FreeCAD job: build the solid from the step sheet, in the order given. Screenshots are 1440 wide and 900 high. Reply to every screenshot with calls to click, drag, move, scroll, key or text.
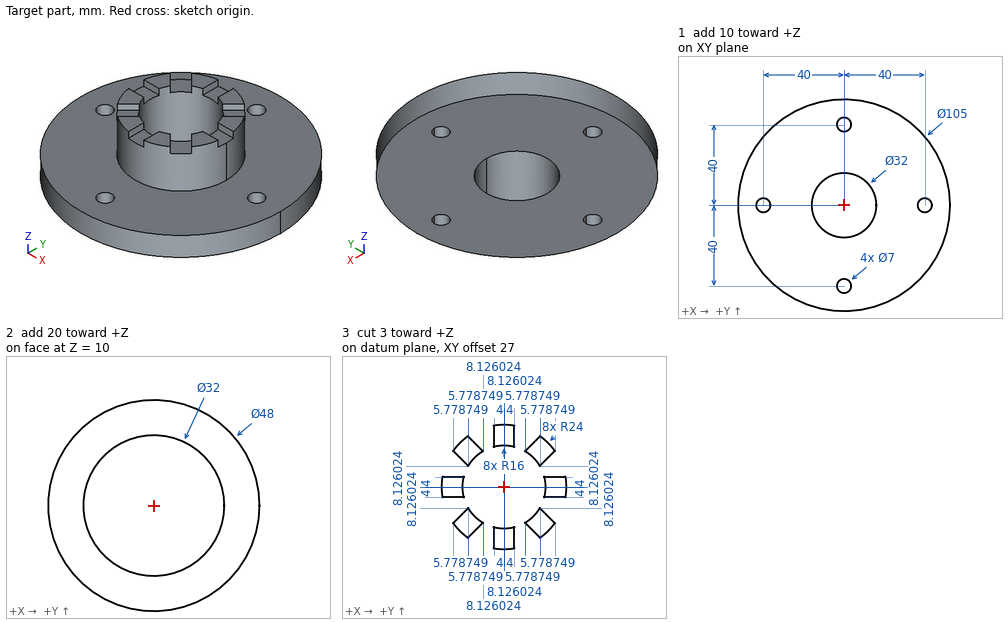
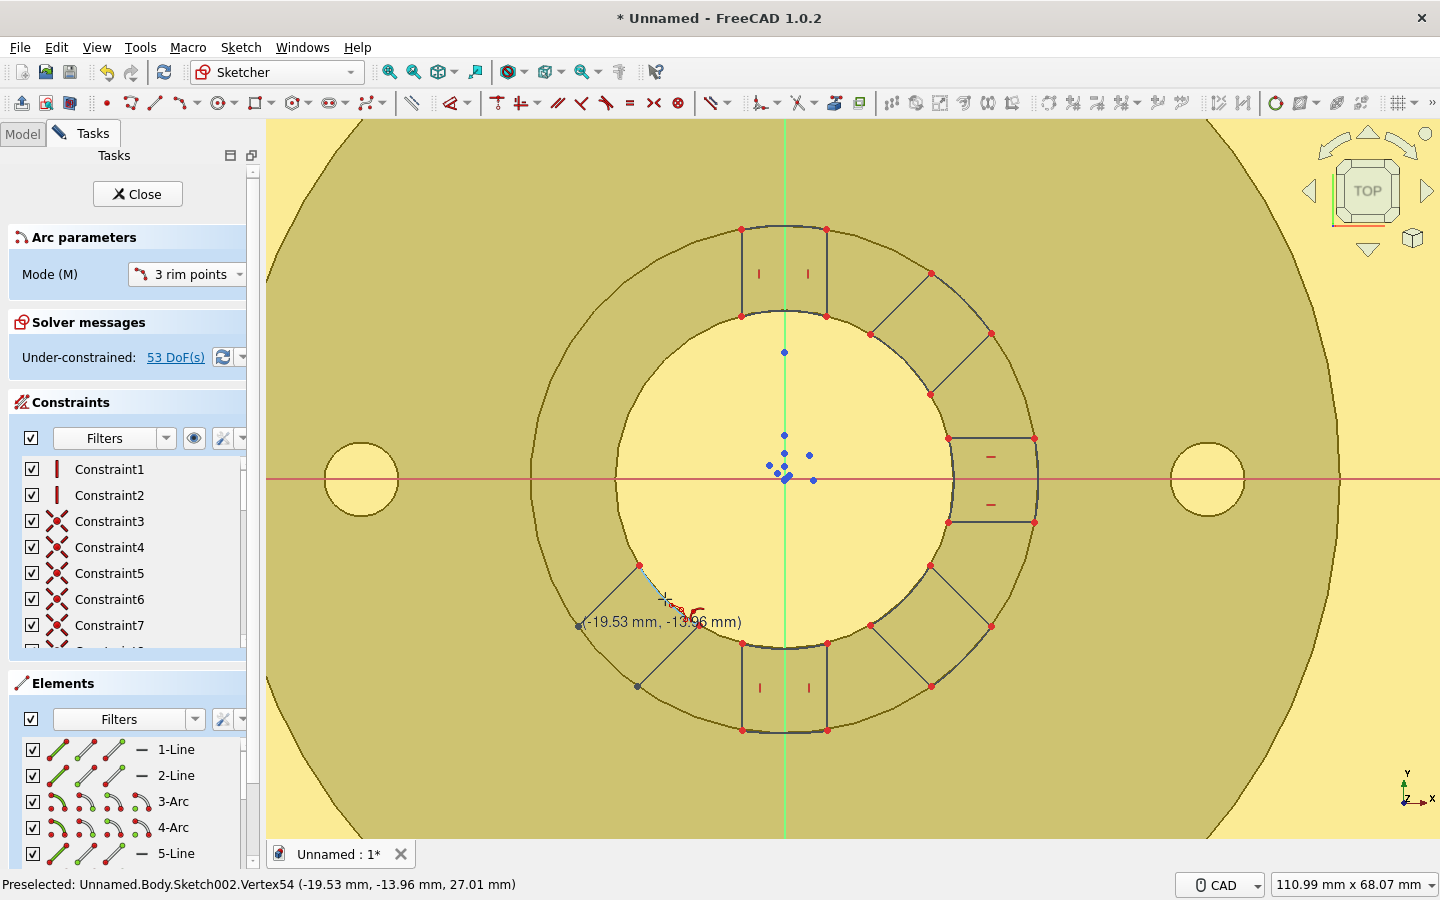
click(637, 687)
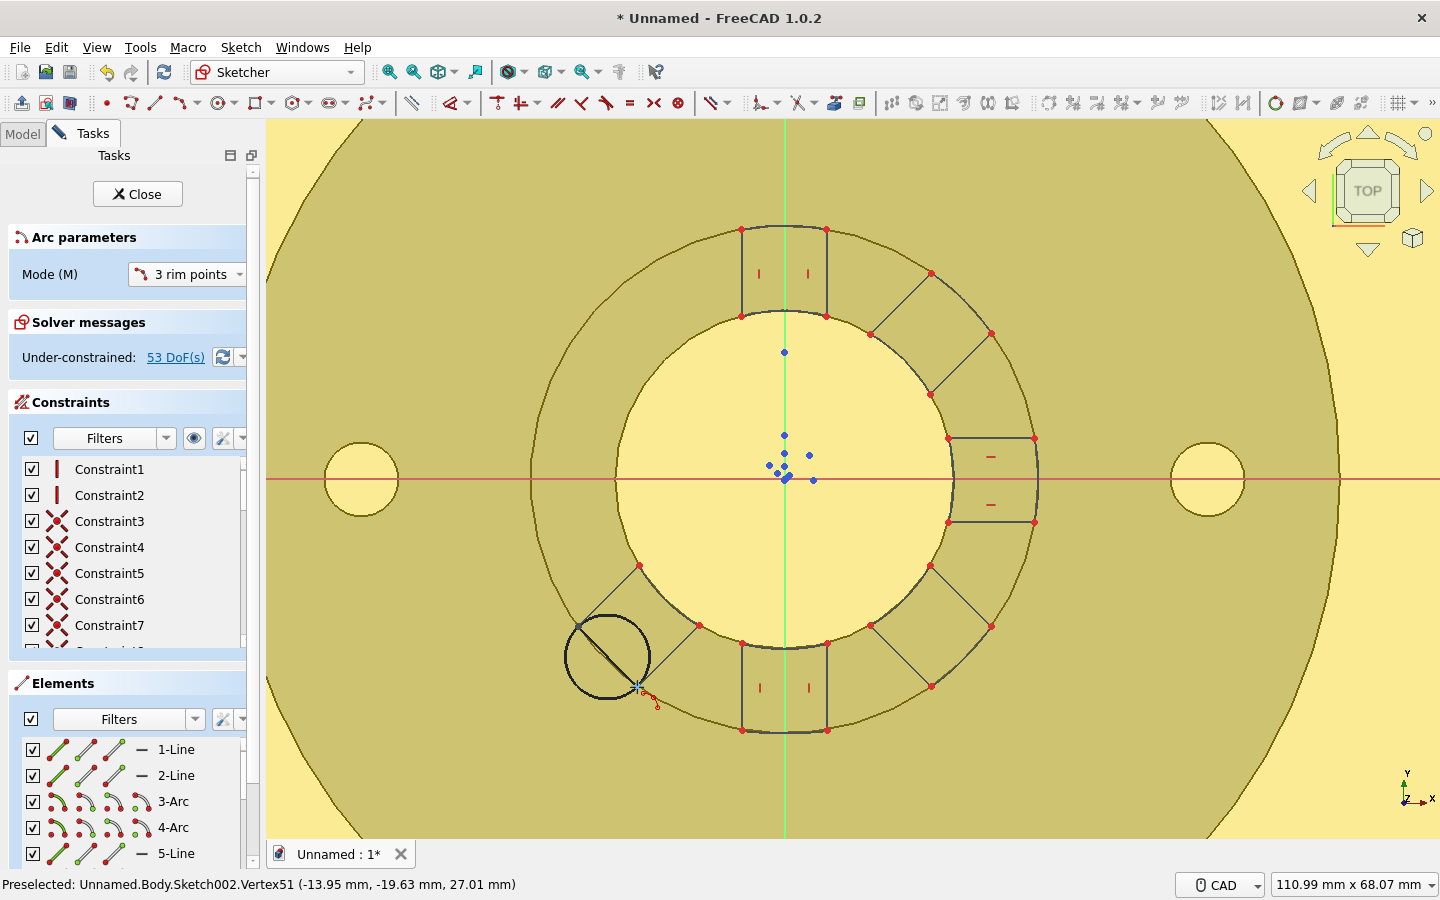
scroll(605, 659, up, 8)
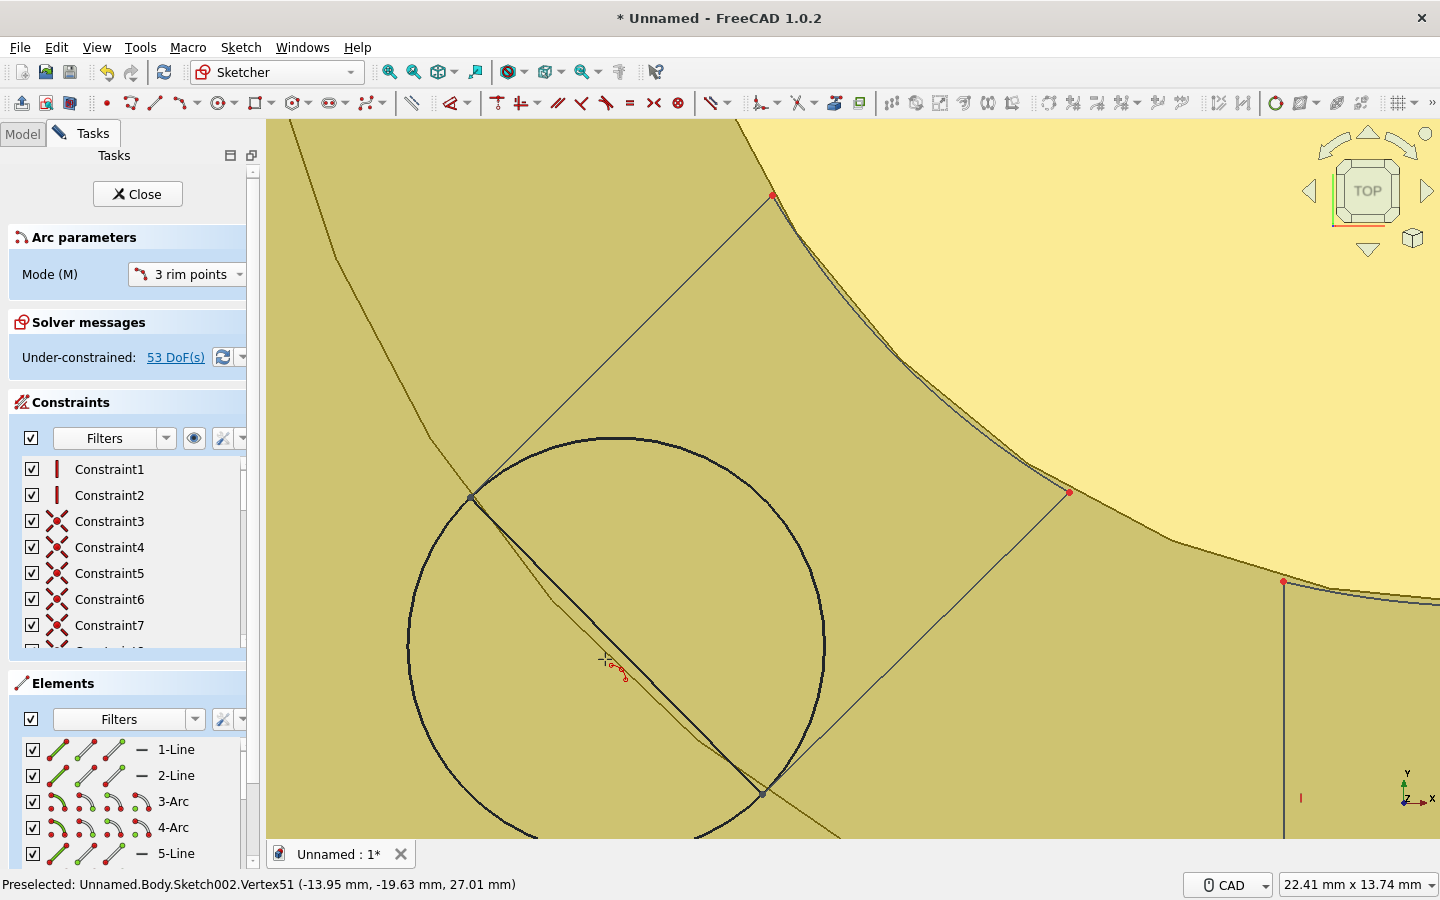
click(604, 655)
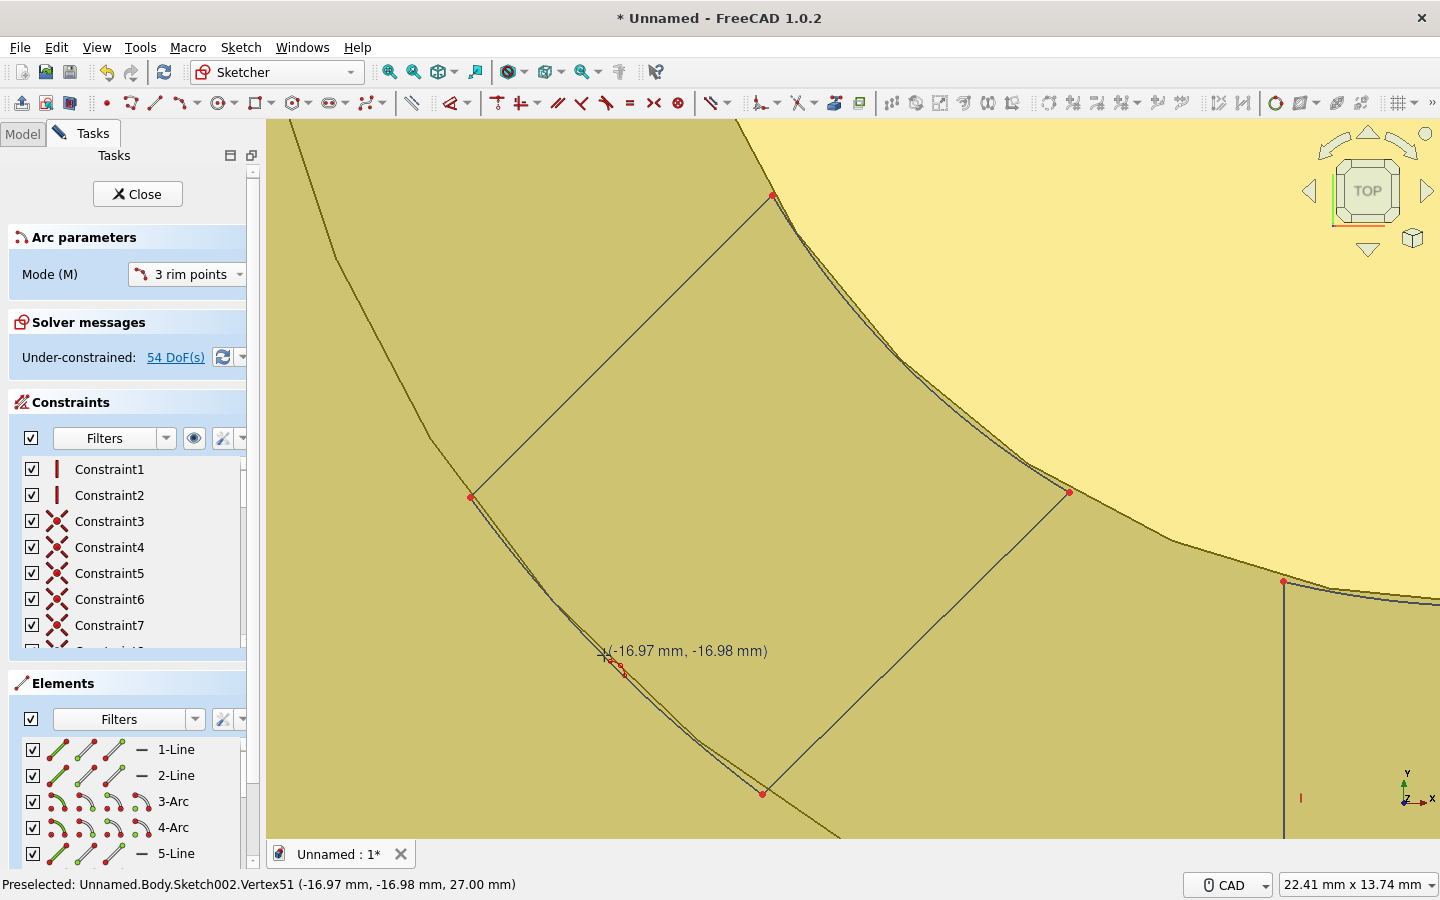
click(156, 104)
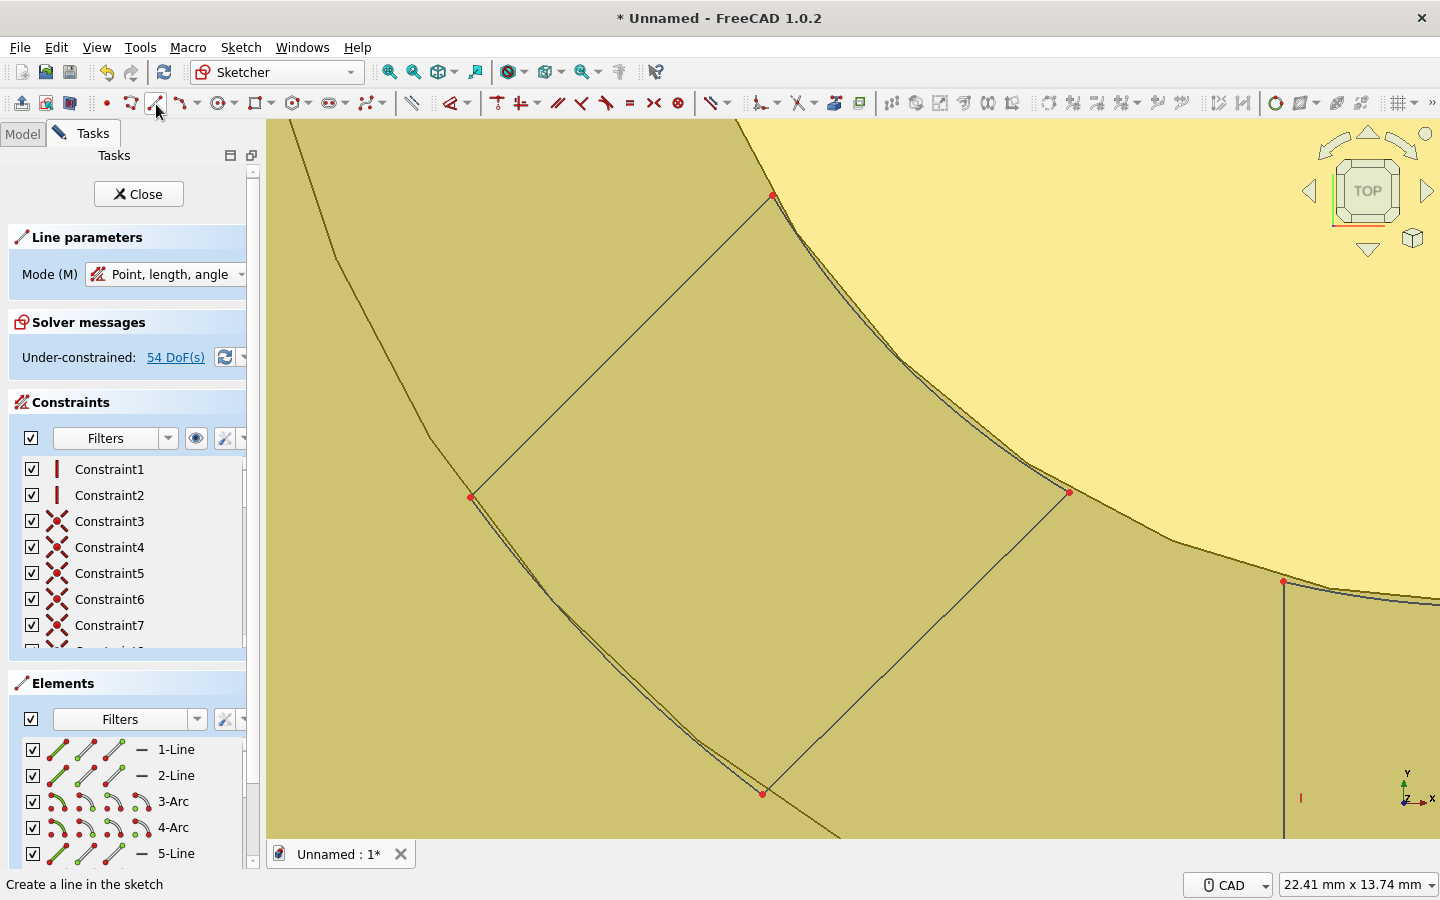
scroll(605, 659, down, 8)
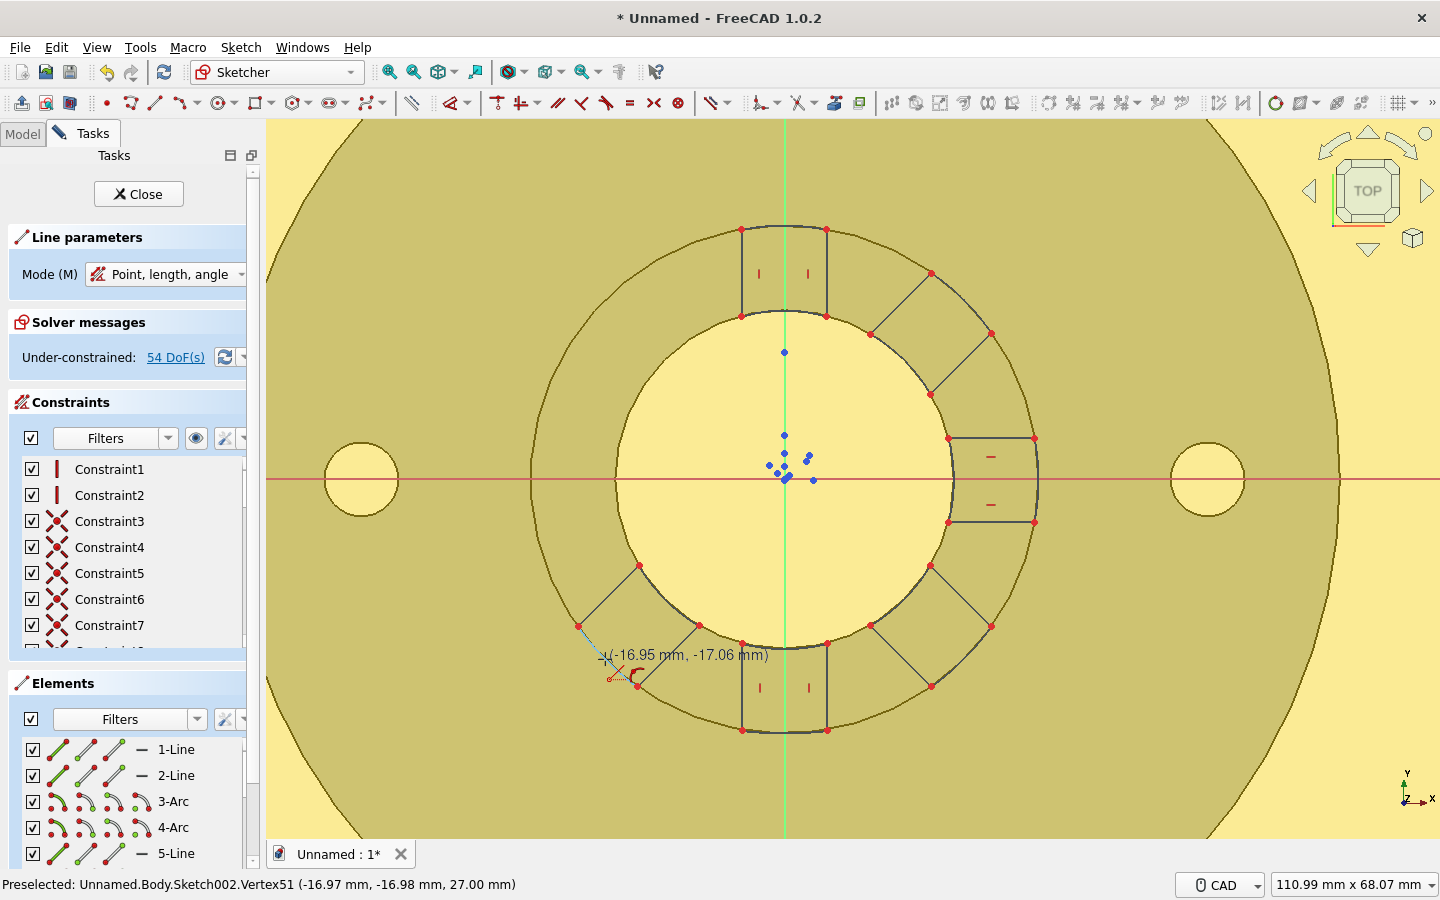
click(534, 522)
click(621, 522)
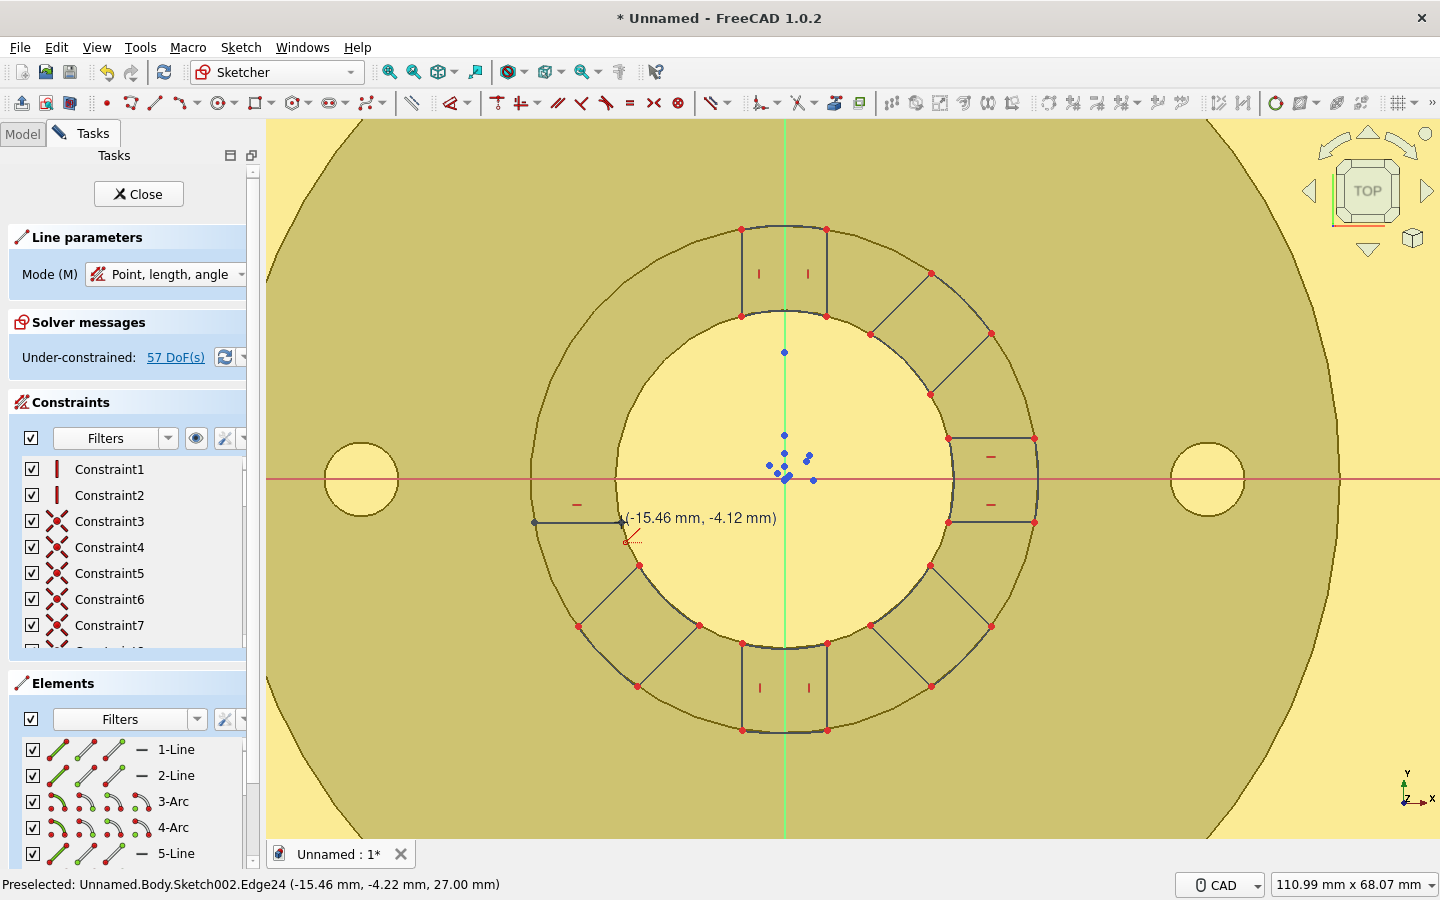
click(621, 437)
click(534, 437)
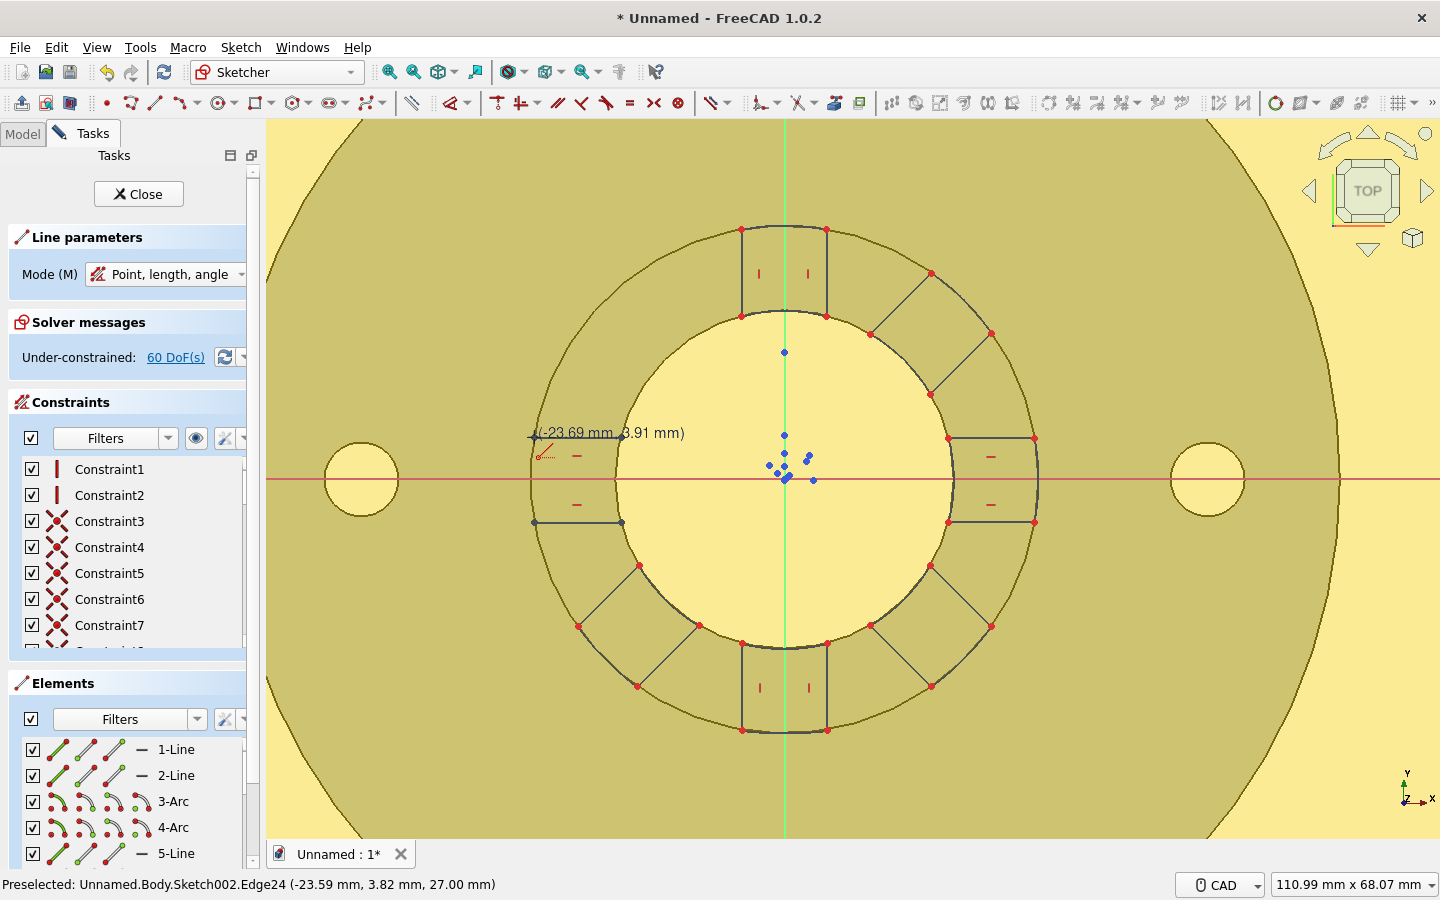
click(180, 104)